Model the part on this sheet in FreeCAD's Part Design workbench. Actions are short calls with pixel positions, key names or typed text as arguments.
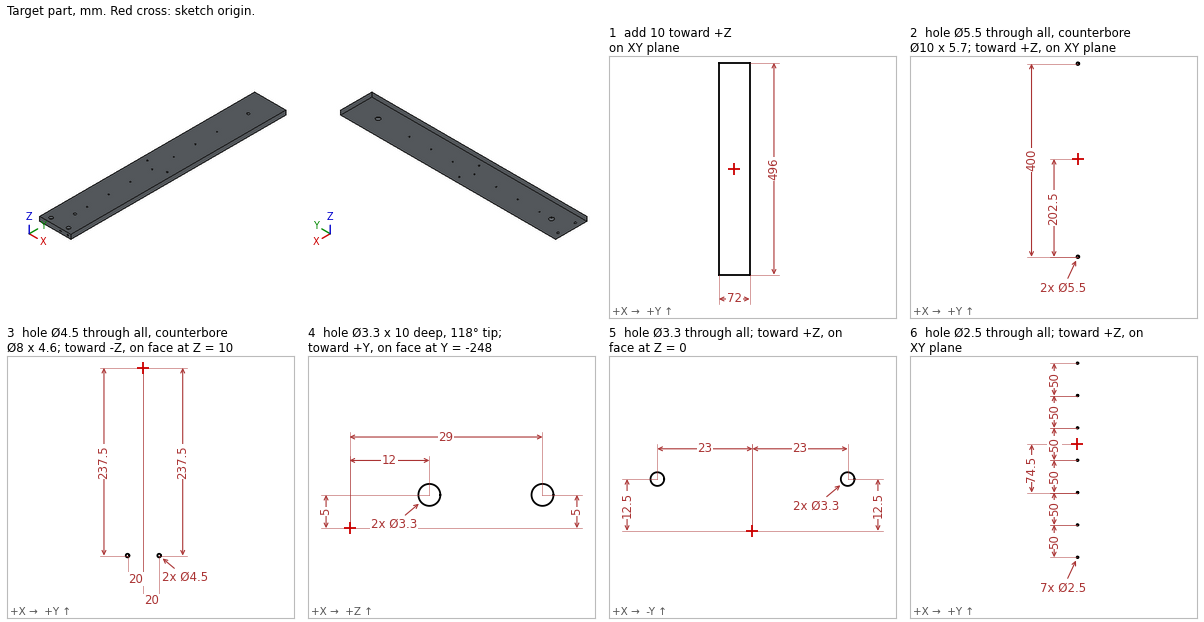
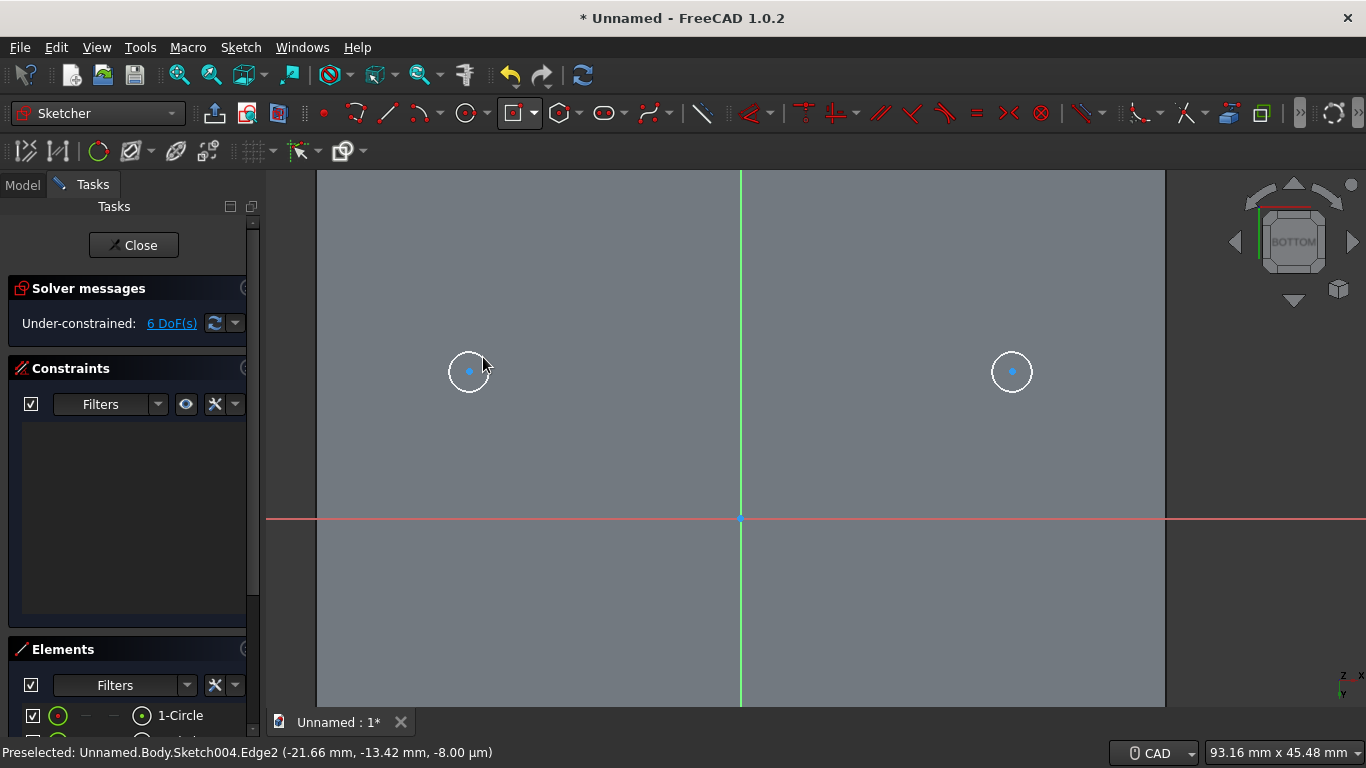
click(1026, 358)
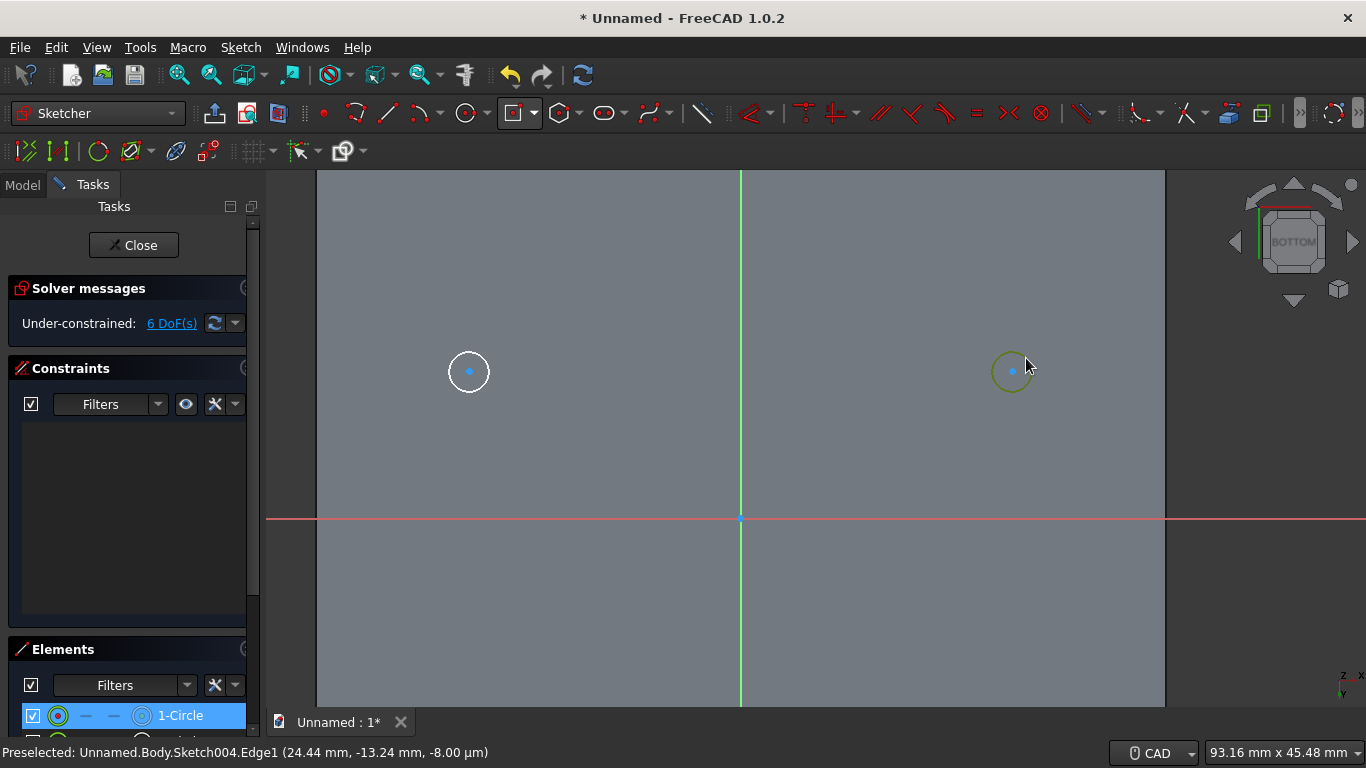
click(483, 358)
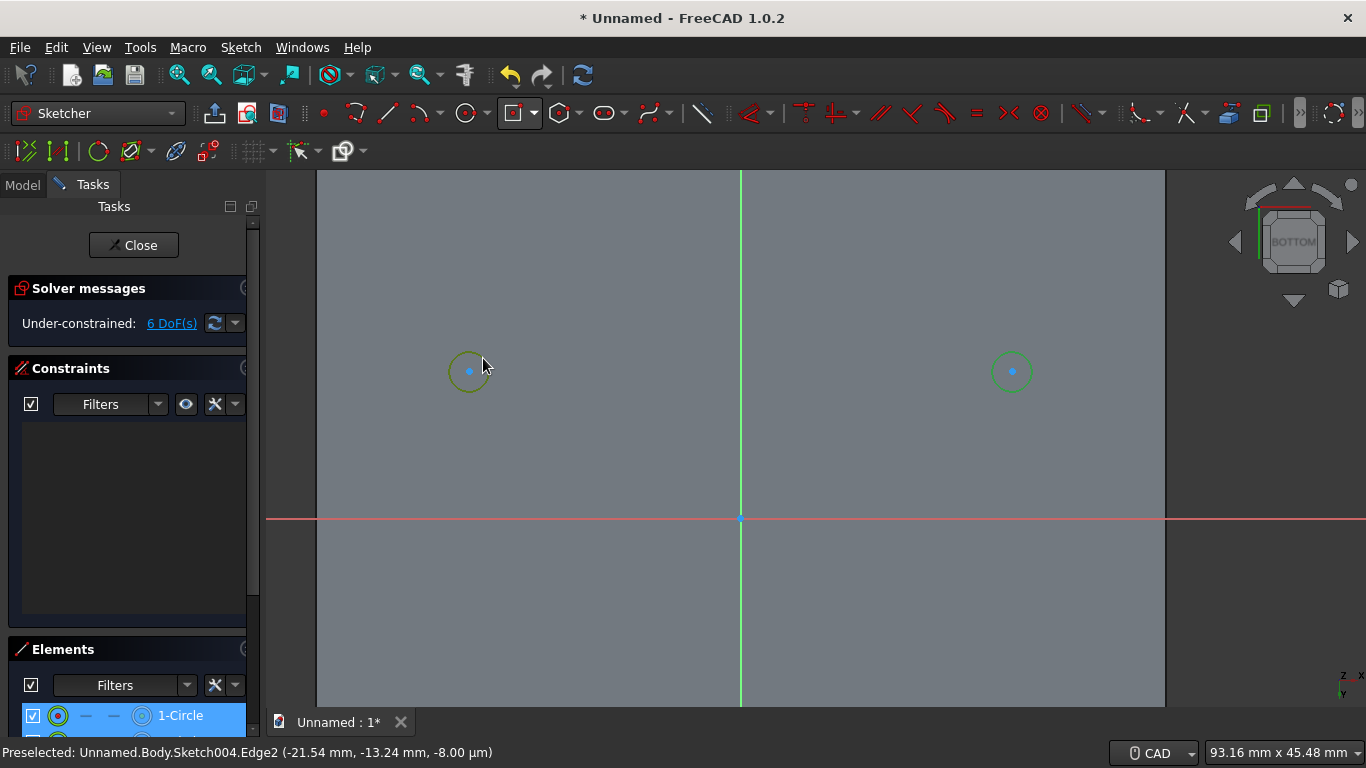
click(978, 114)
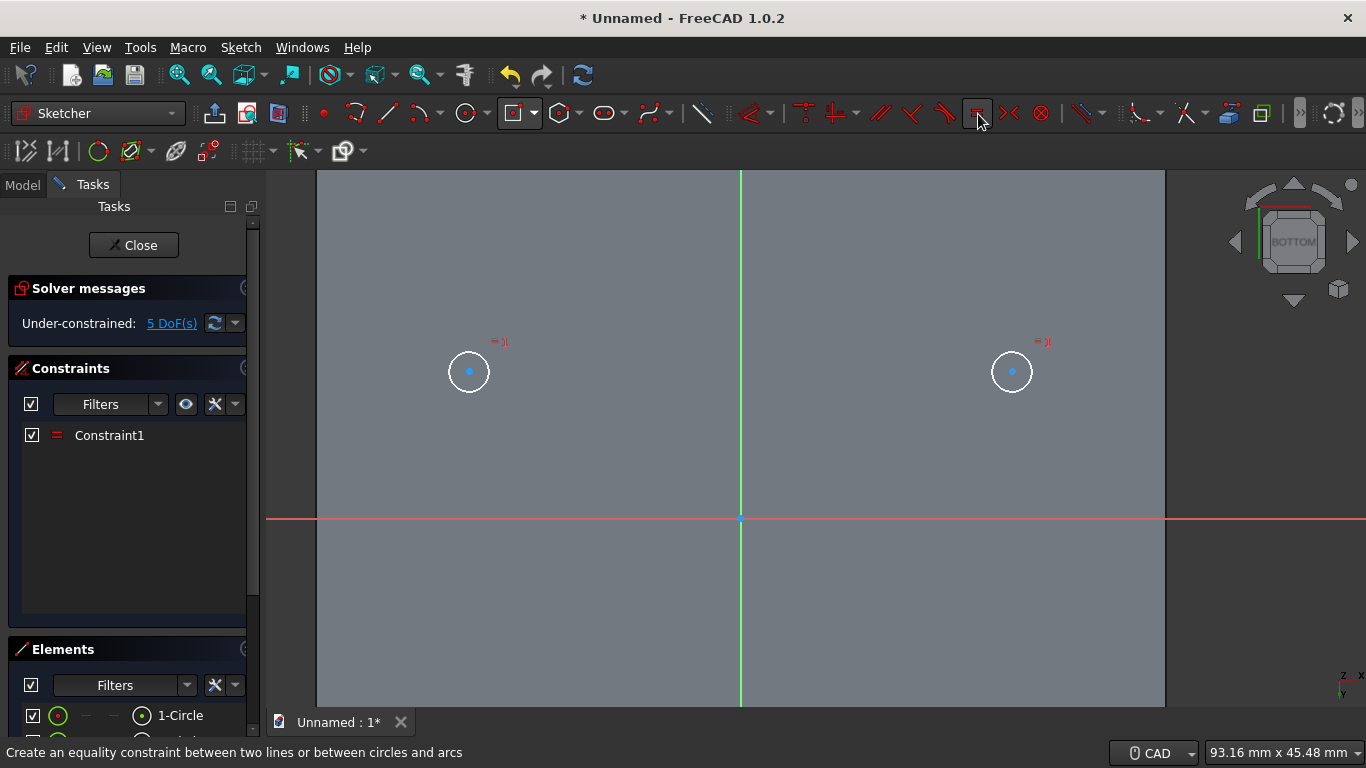
click(750, 114)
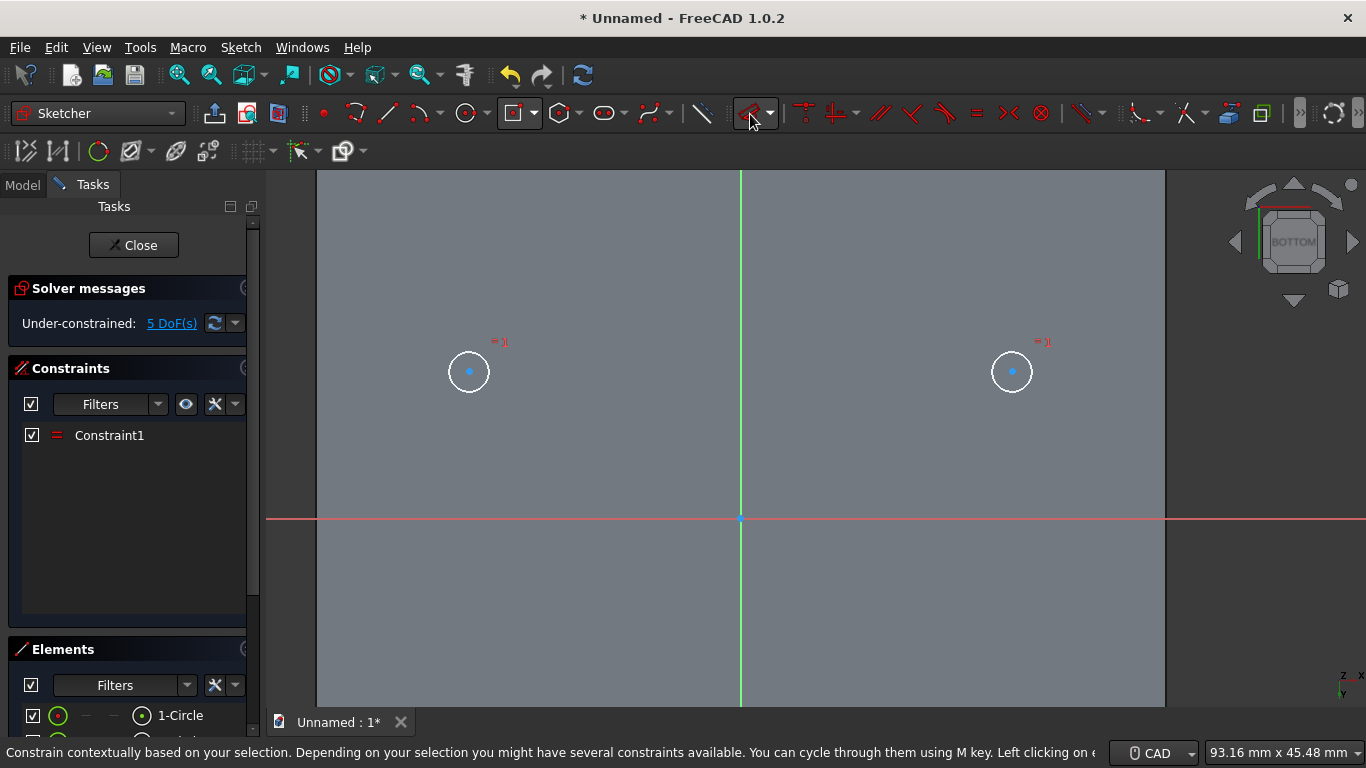
click(1026, 358)
click(1049, 335)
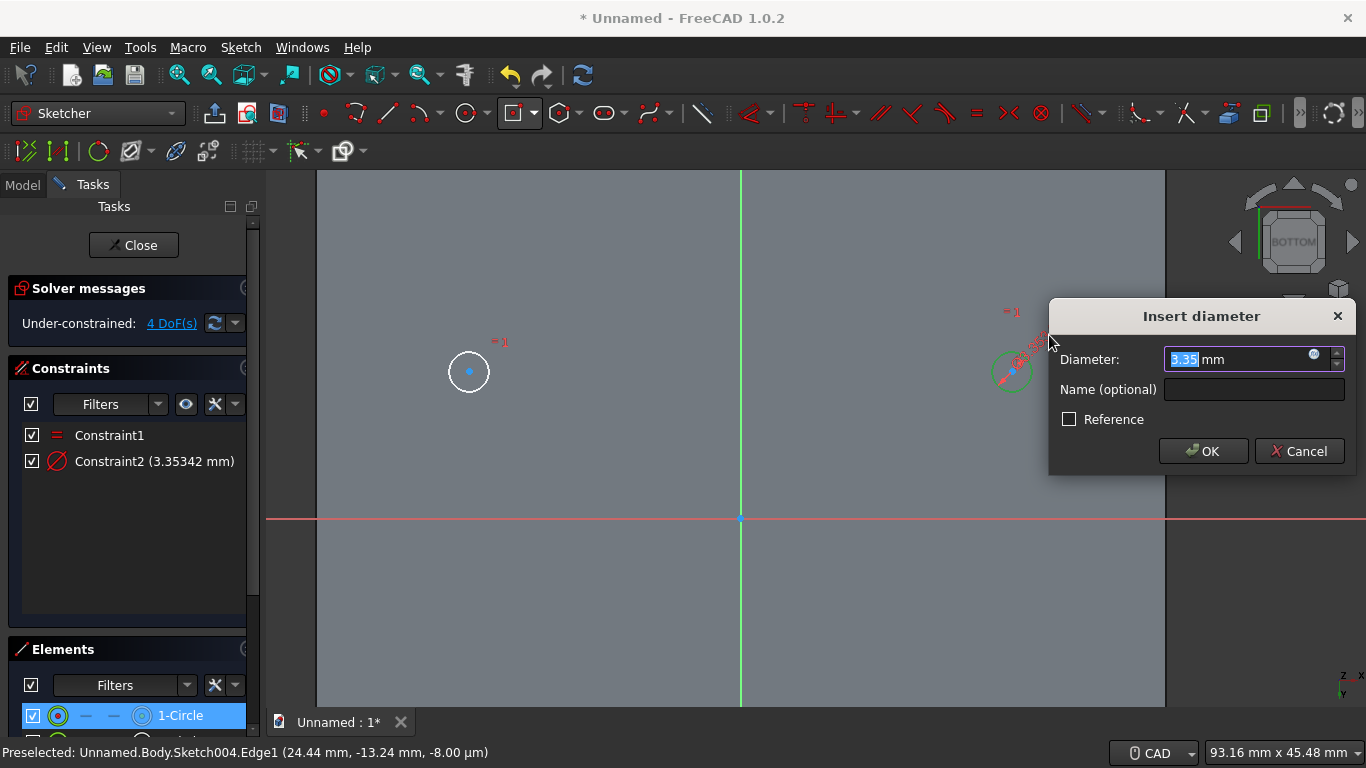
text(3.3)
key(Return)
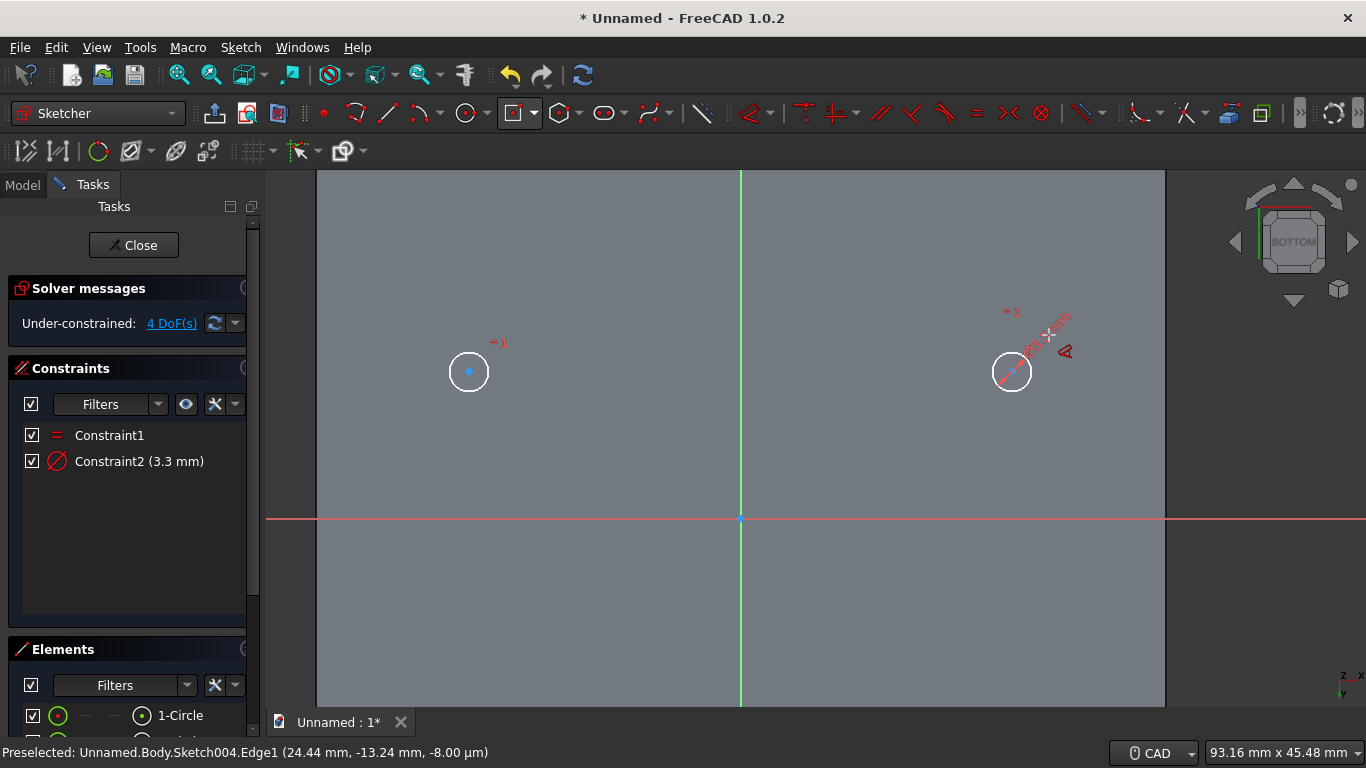
click(1012, 372)
click(876, 553)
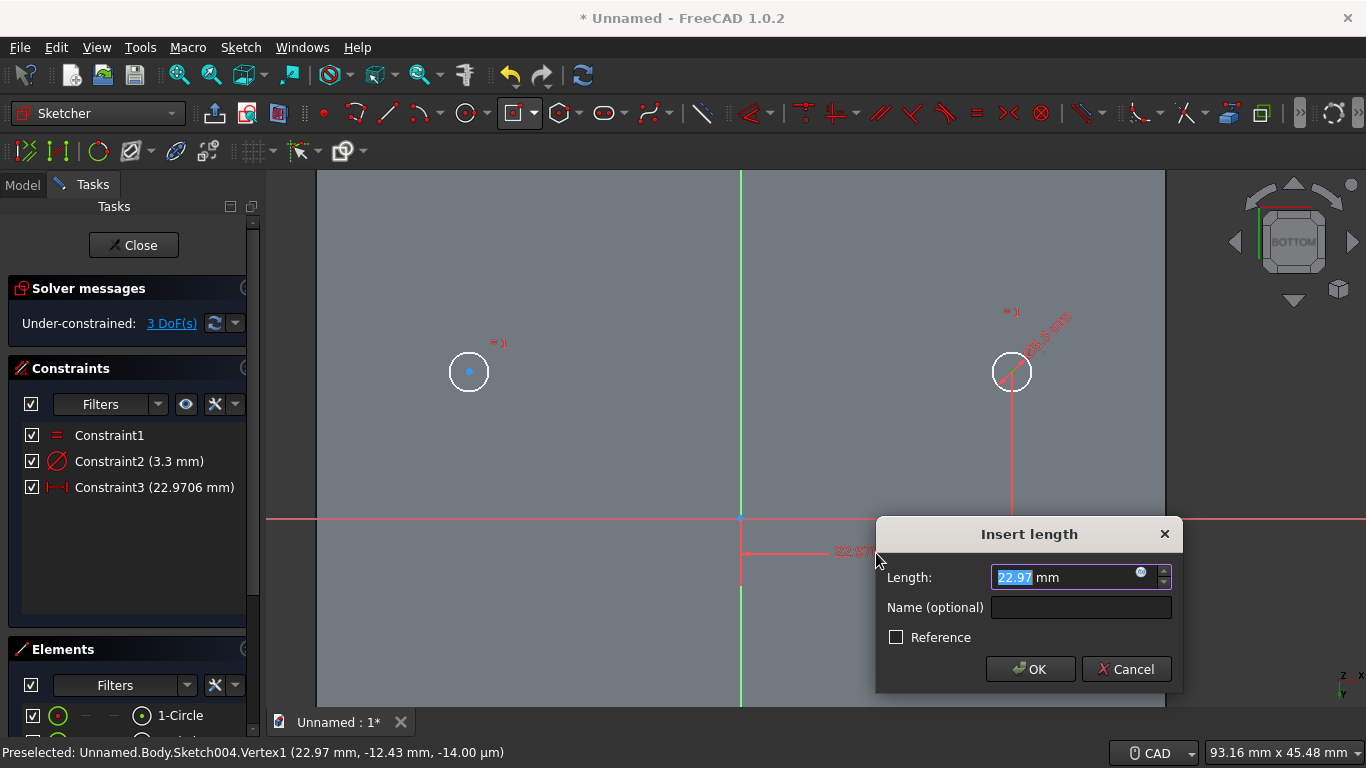
text(23)
key(Return)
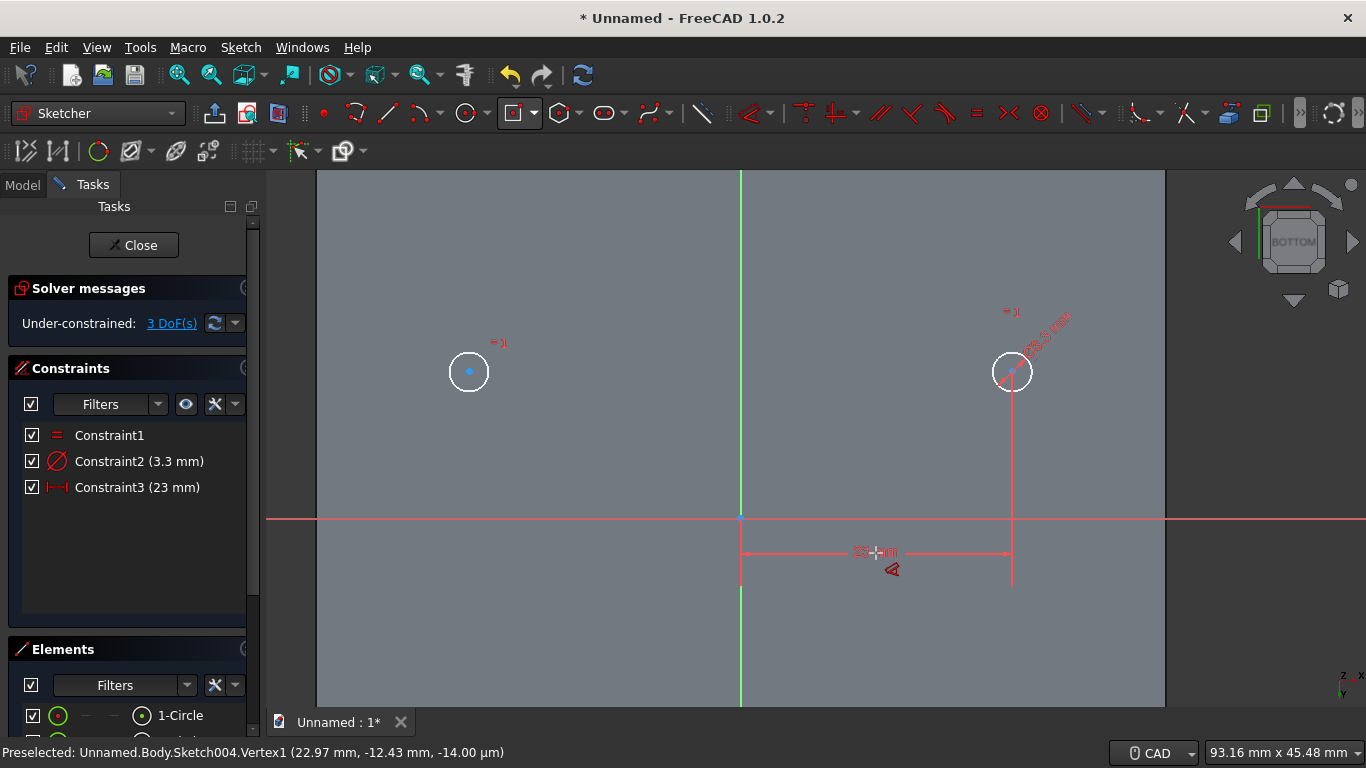
click(469, 372)
click(605, 553)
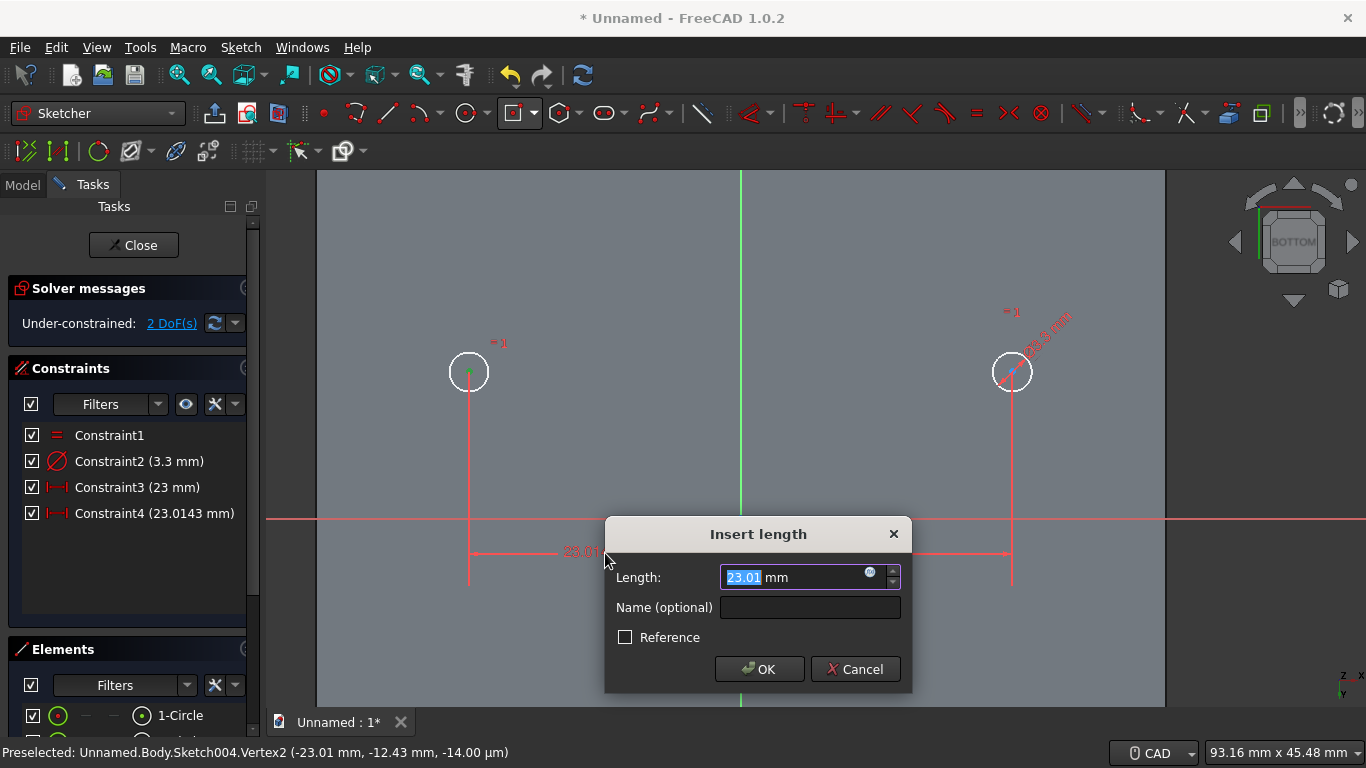
text(23)
key(Return)